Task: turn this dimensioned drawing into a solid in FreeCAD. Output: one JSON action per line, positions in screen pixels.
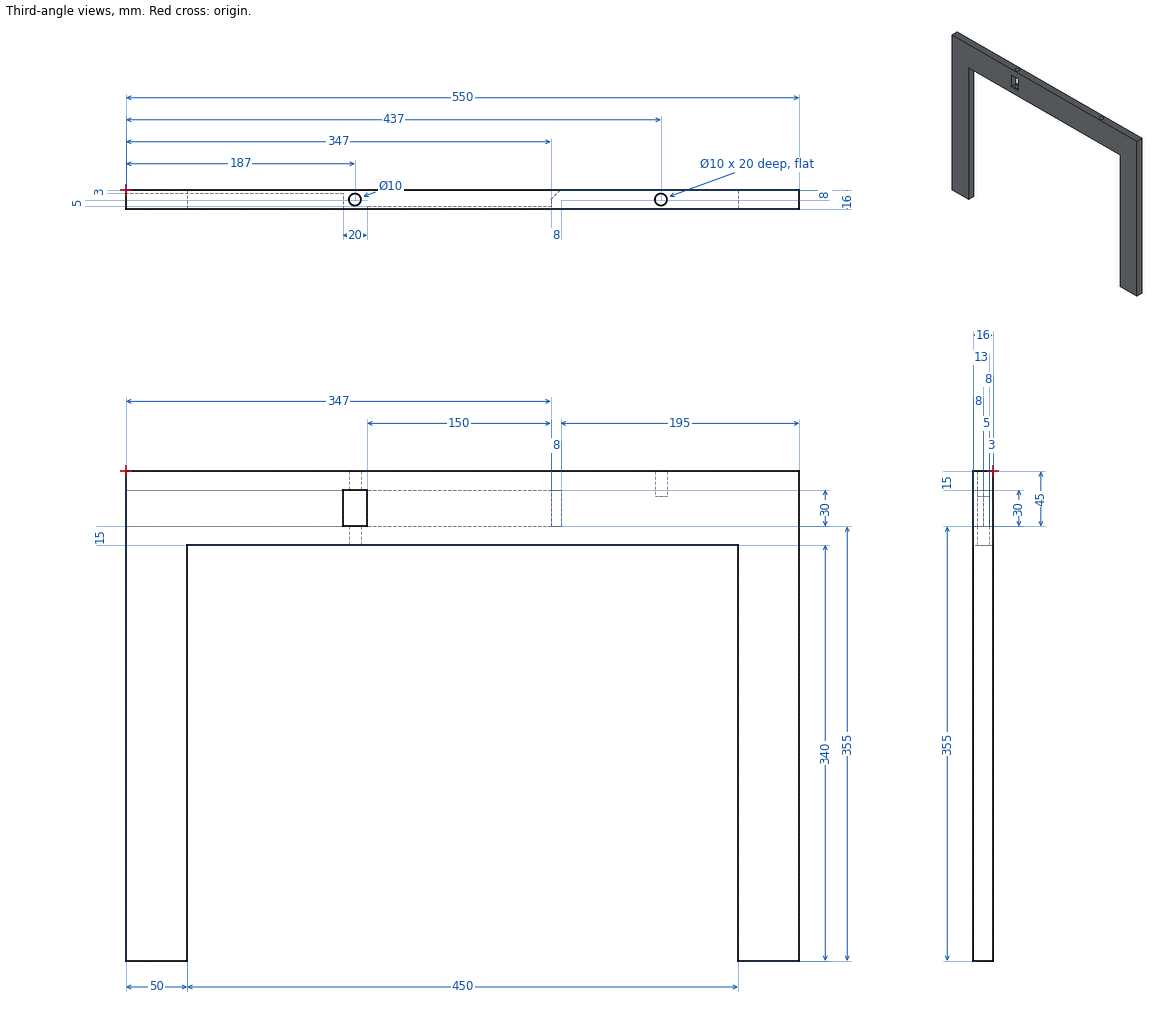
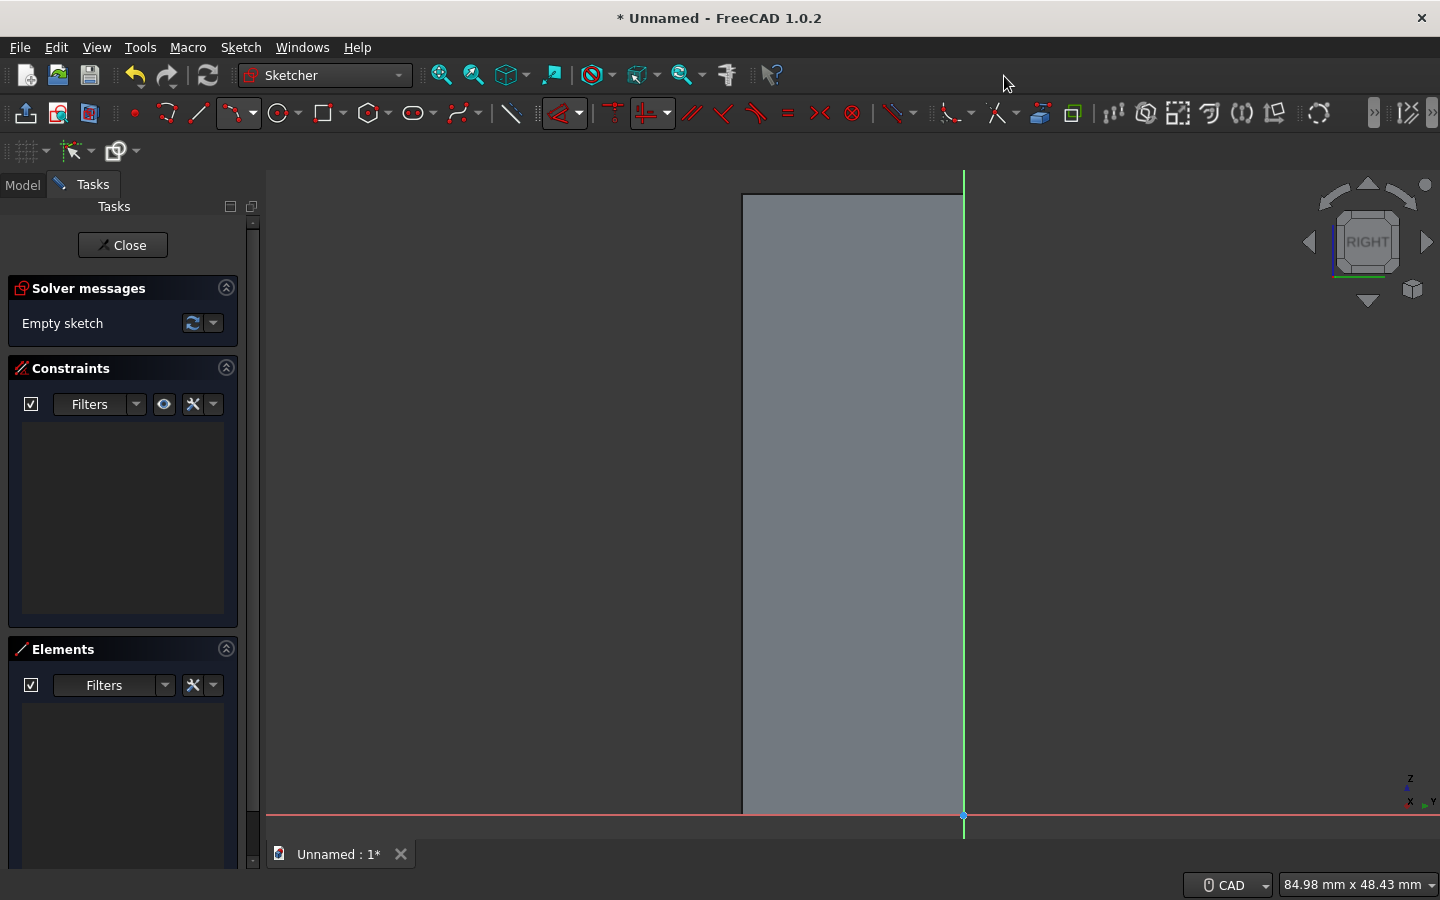
{"action": "scroll", "coordinate": [645, 504], "scroll_direction": "down", "scroll_amount": 2}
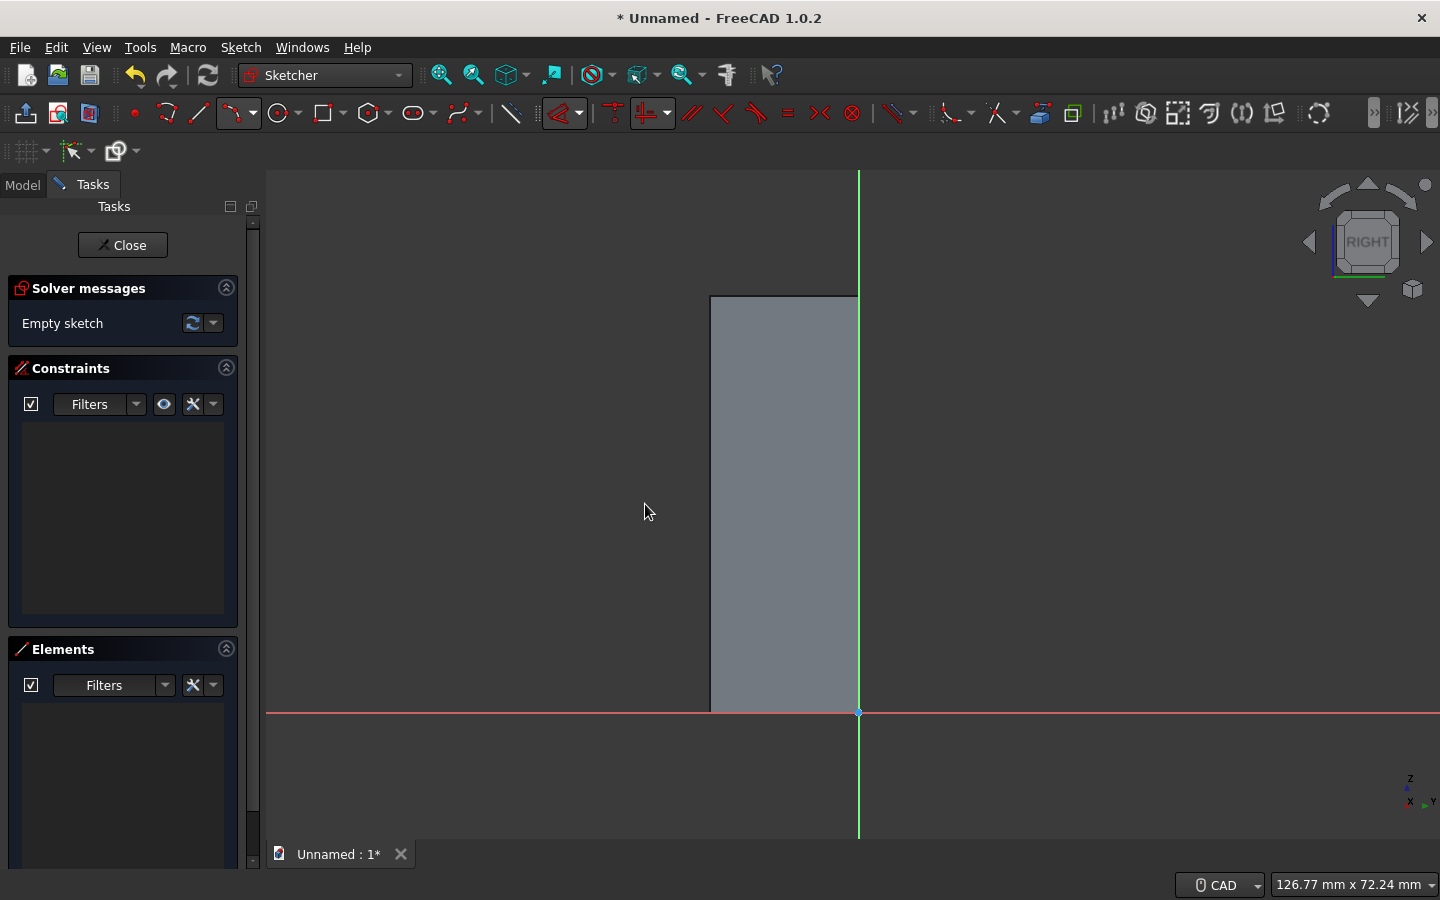
{"action": "left_click", "coordinate": [324, 114]}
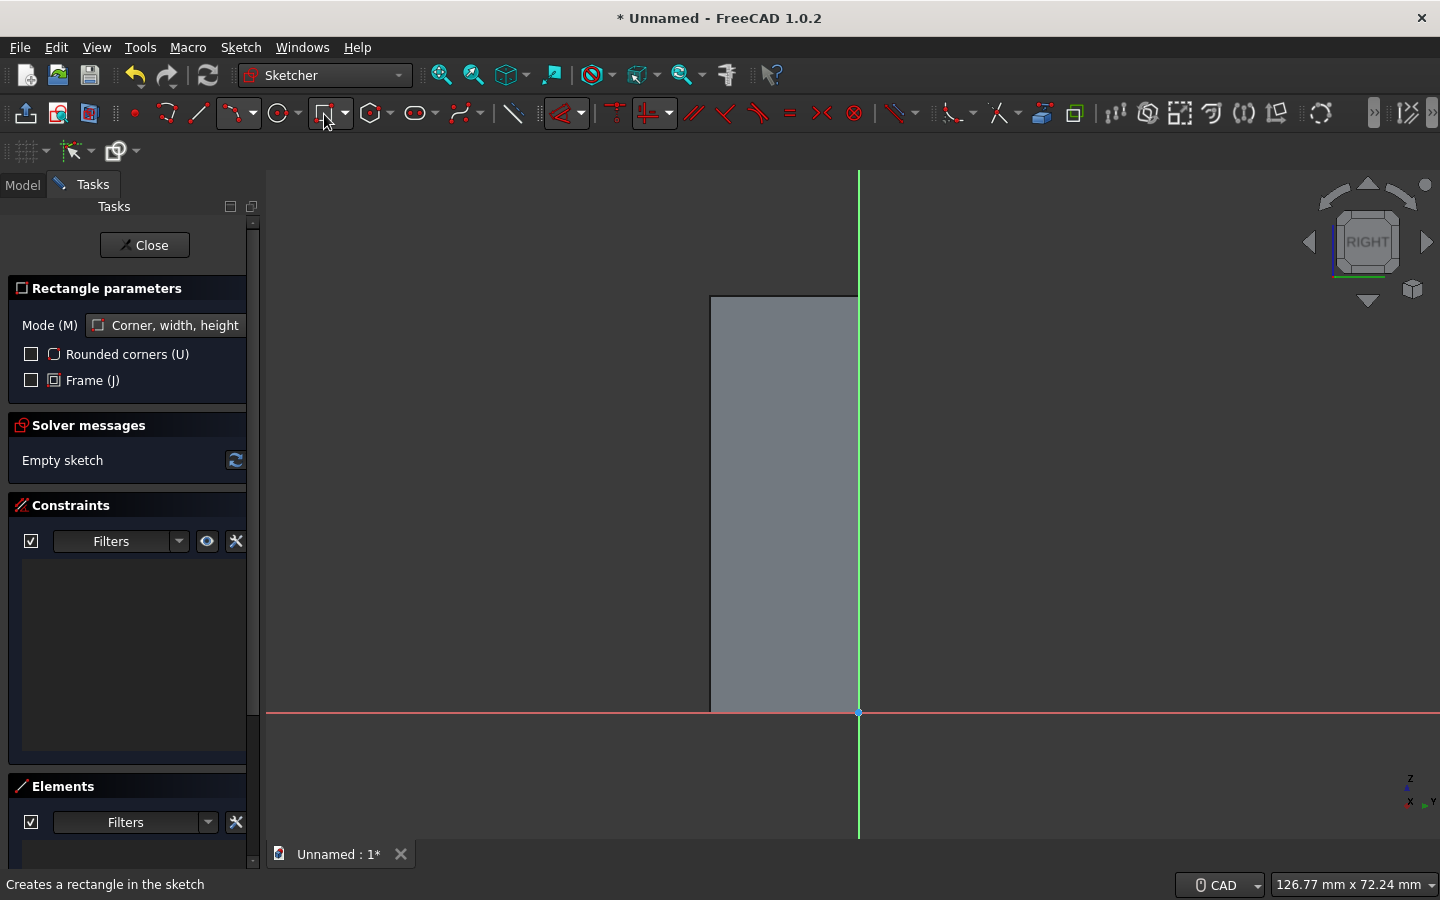
{"action": "left_click", "coordinate": [859, 713]}
{"action": "left_click", "coordinate": [710, 296]}
{"action": "key", "text": "Escape"}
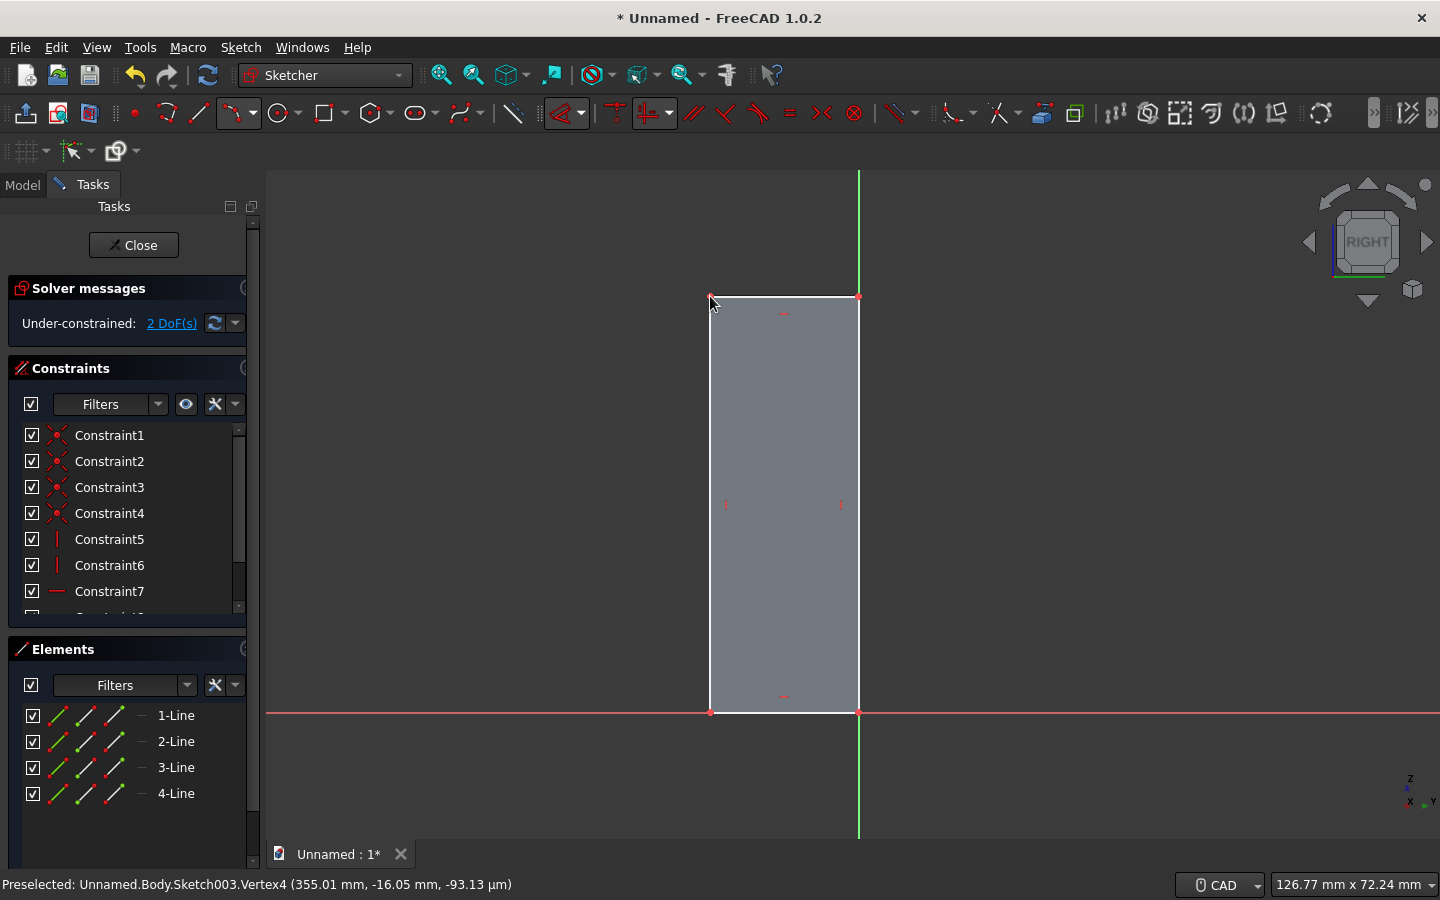
{"action": "left_click", "coordinate": [859, 588]}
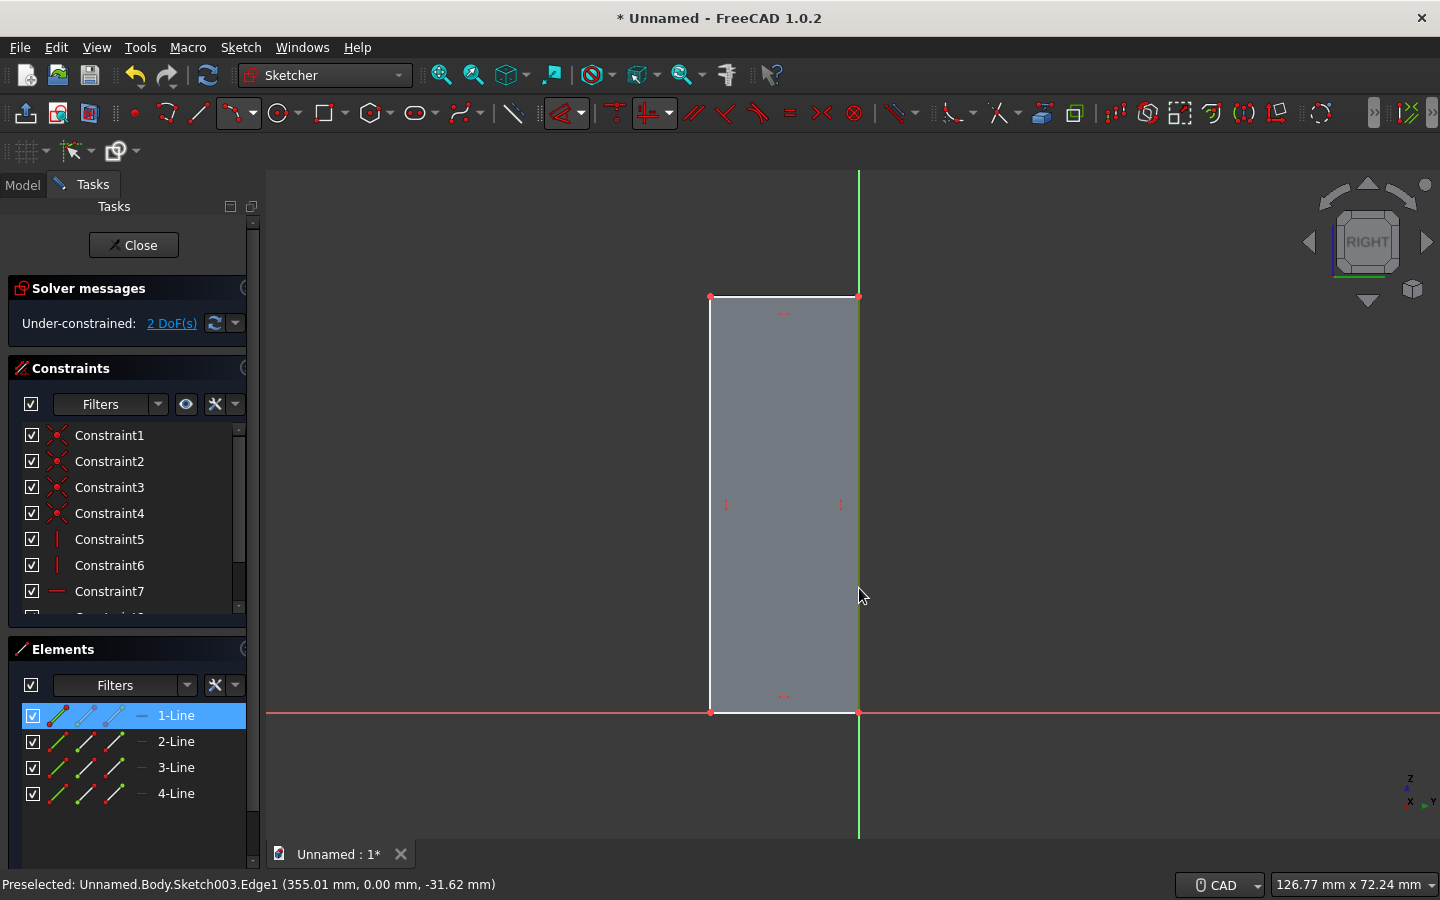
{"action": "left_click", "coordinate": [584, 114]}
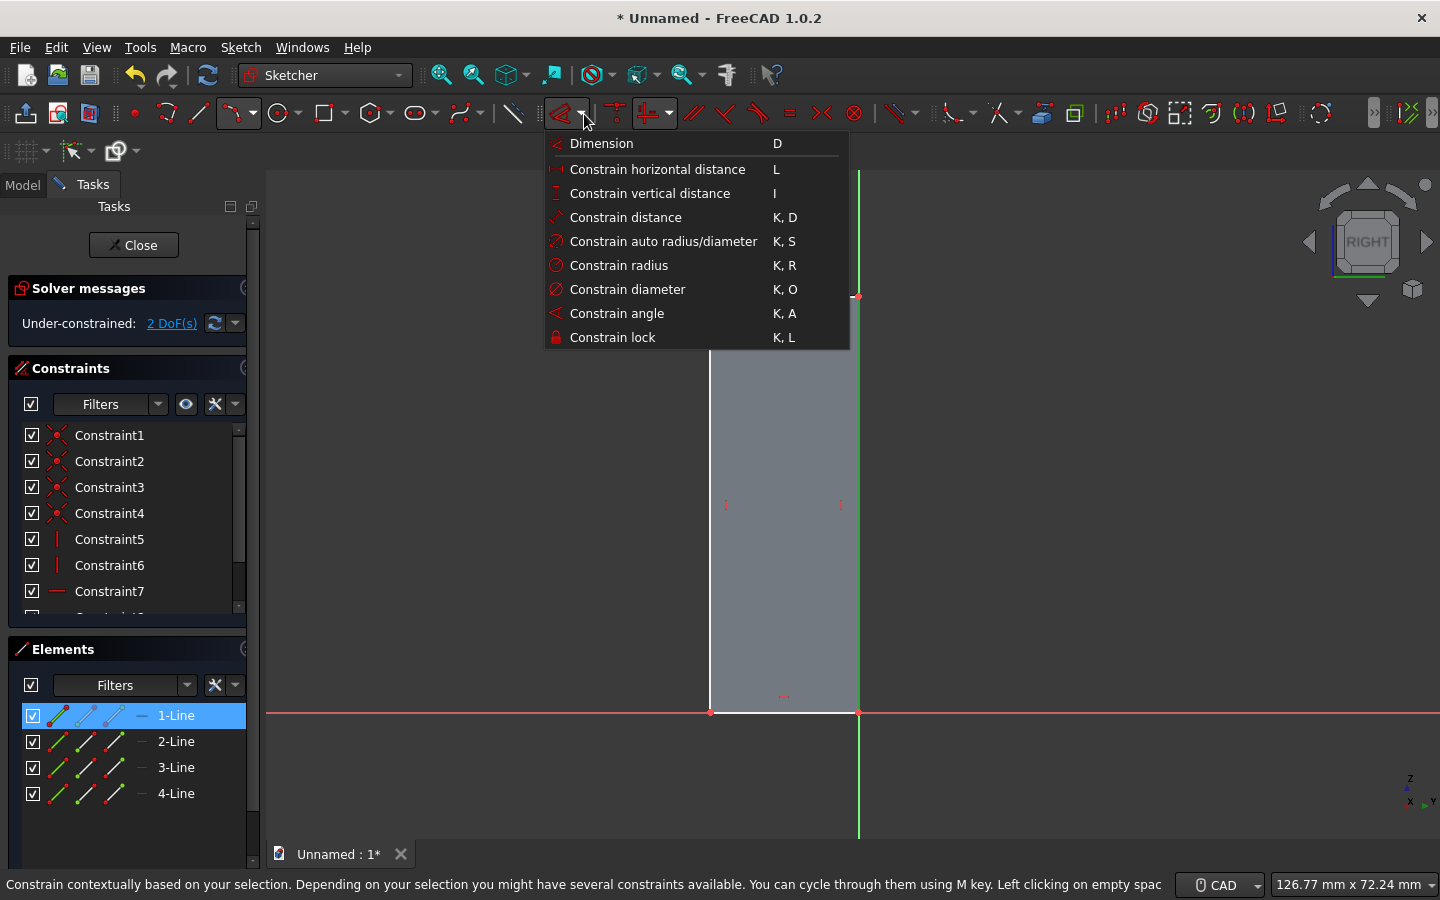
{"action": "left_click", "coordinate": [697, 193]}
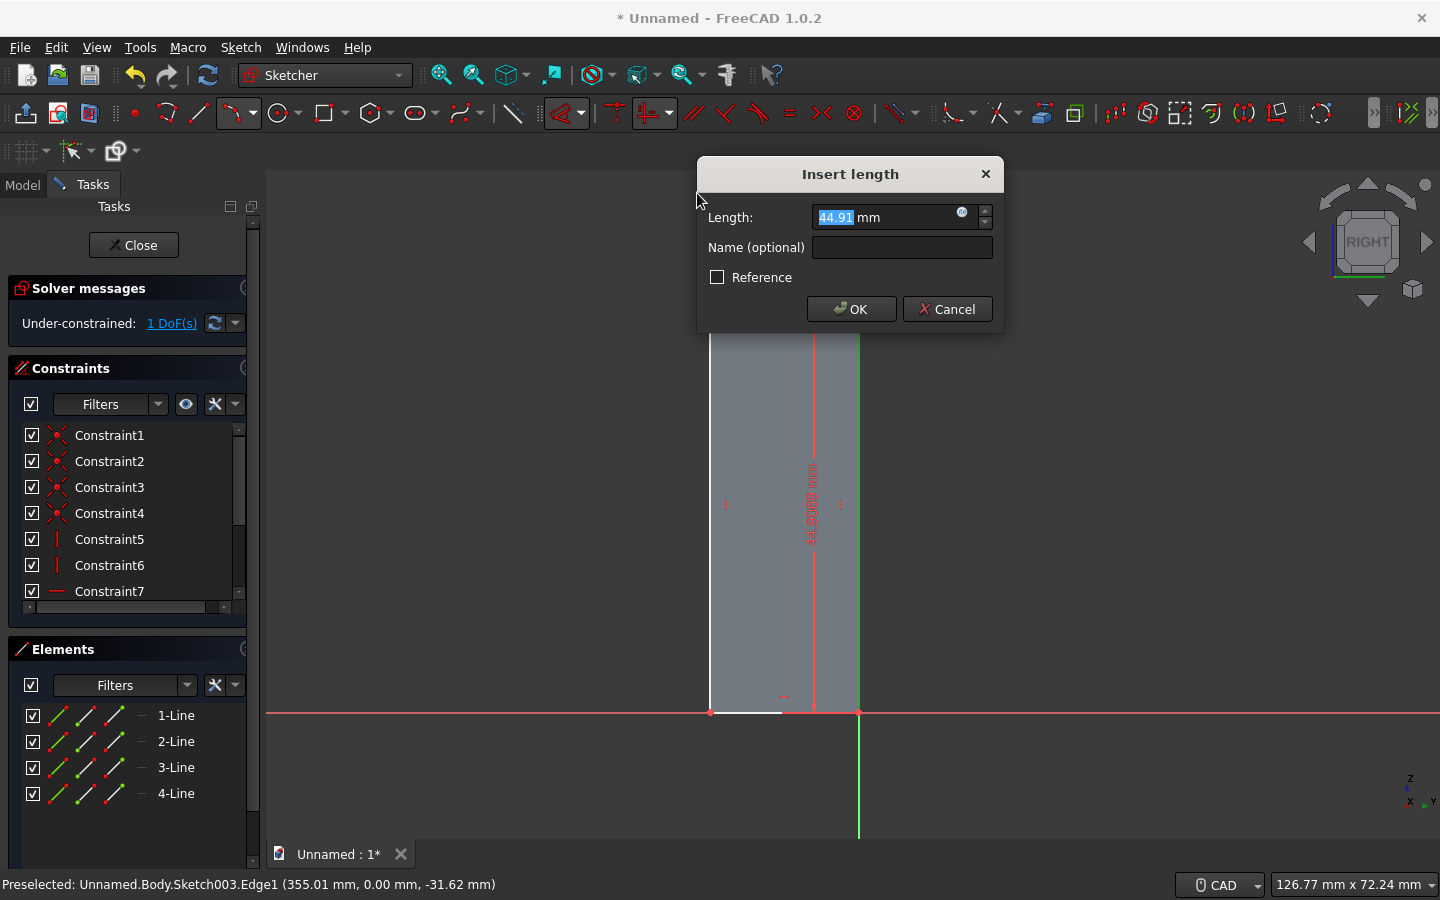
{"action": "type", "text": "45"}
{"action": "key", "text": "Return"}